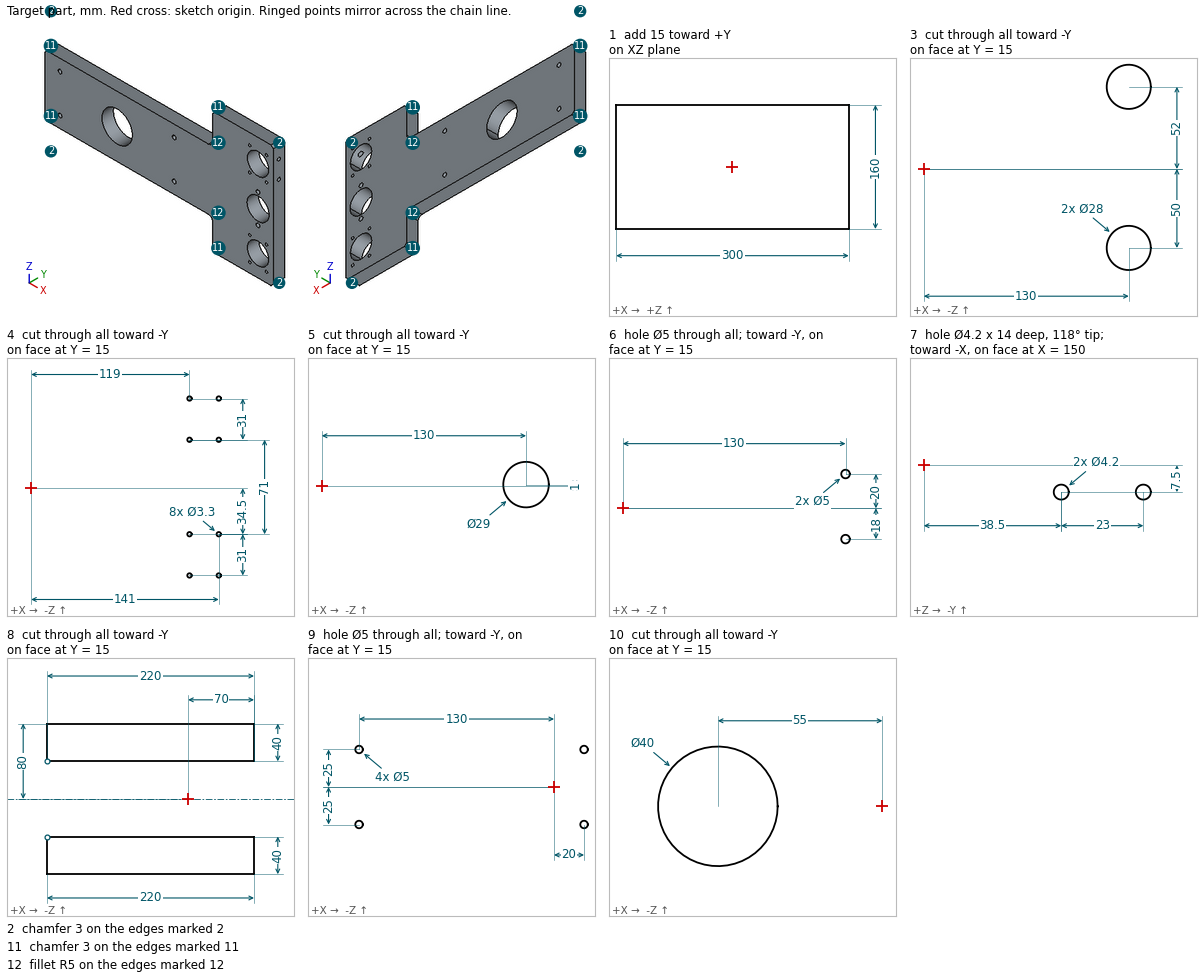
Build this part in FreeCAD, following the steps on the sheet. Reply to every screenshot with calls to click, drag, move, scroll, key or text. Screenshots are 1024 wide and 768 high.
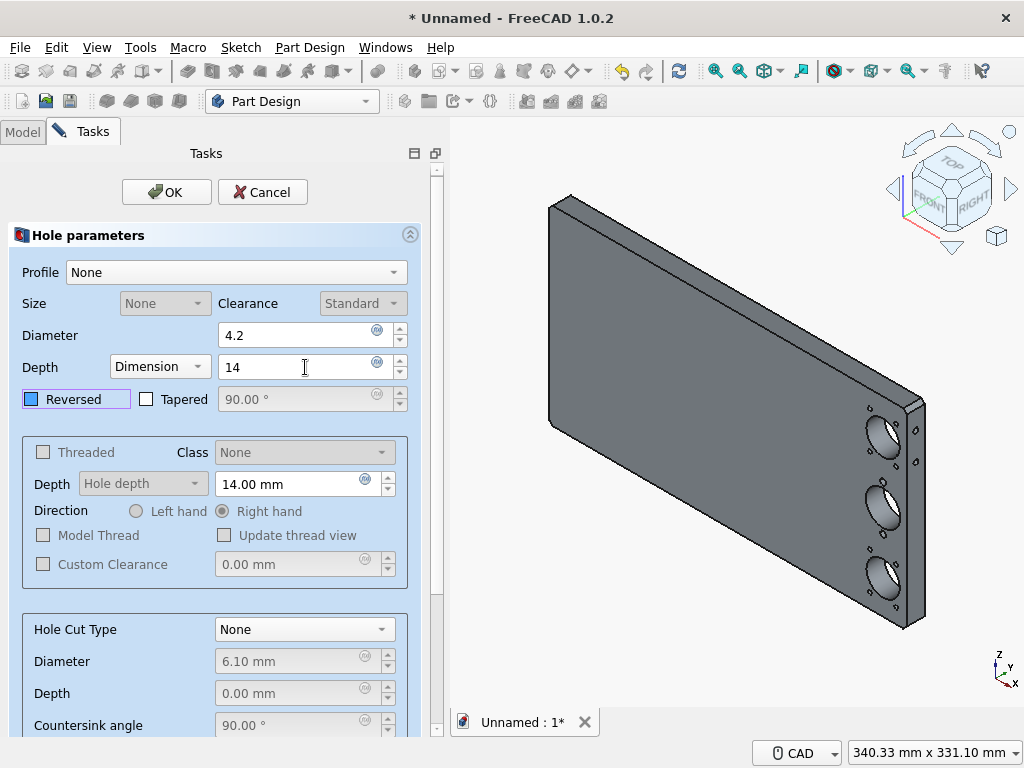
click(167, 192)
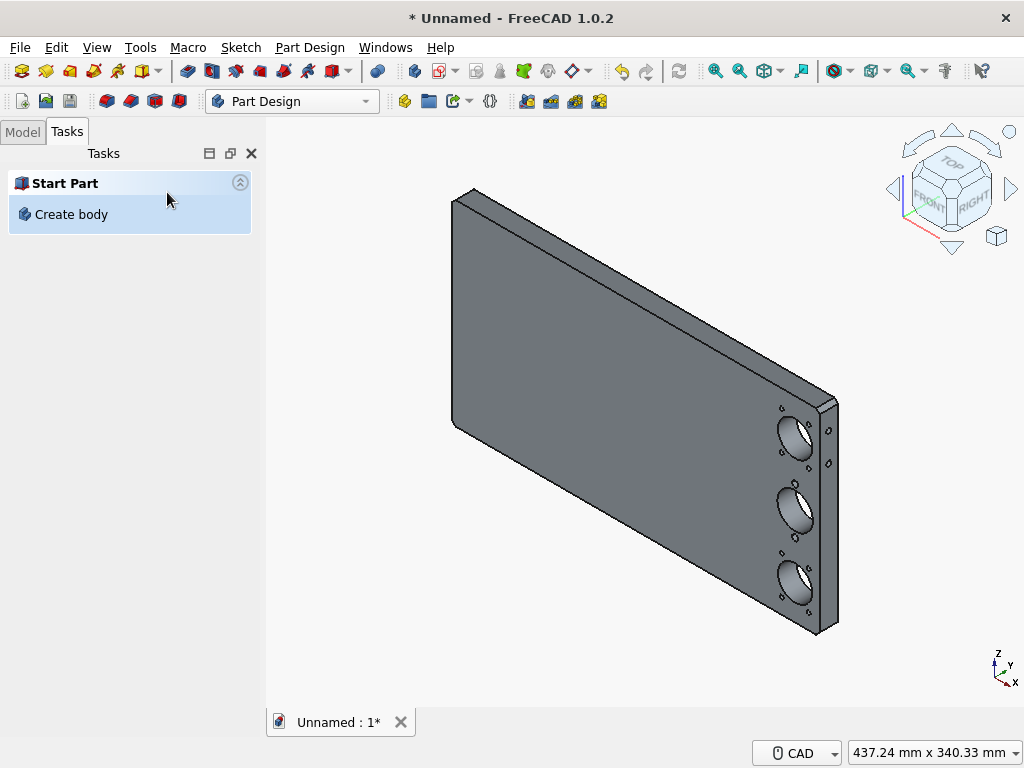
key(4)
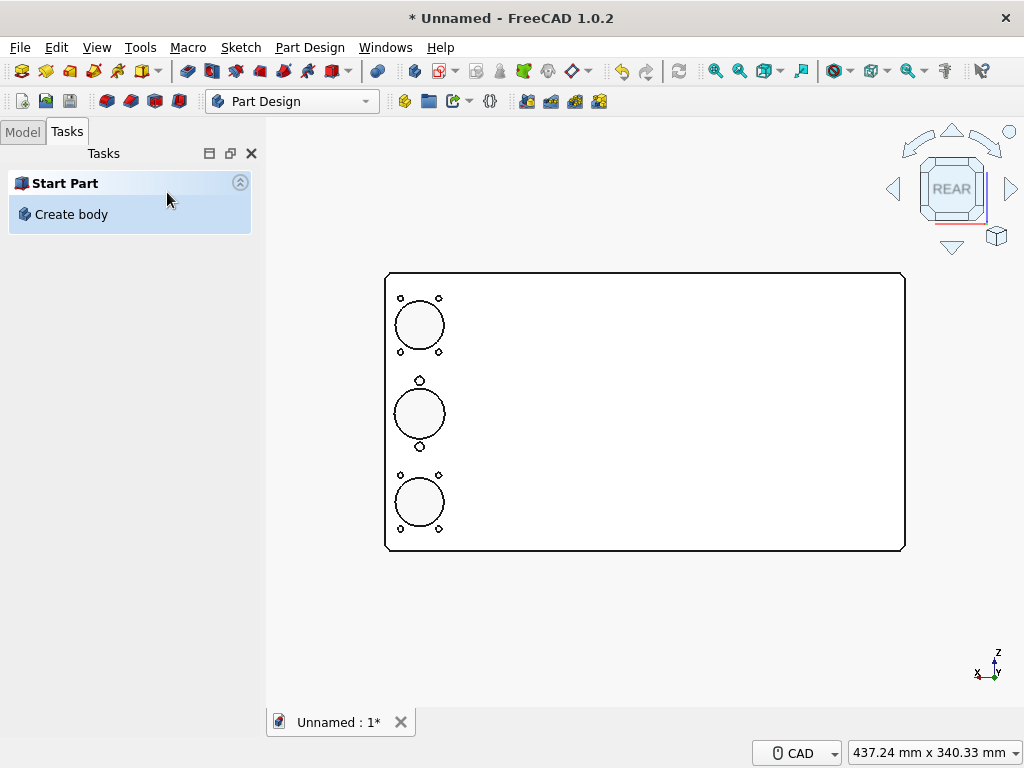
click(645, 411)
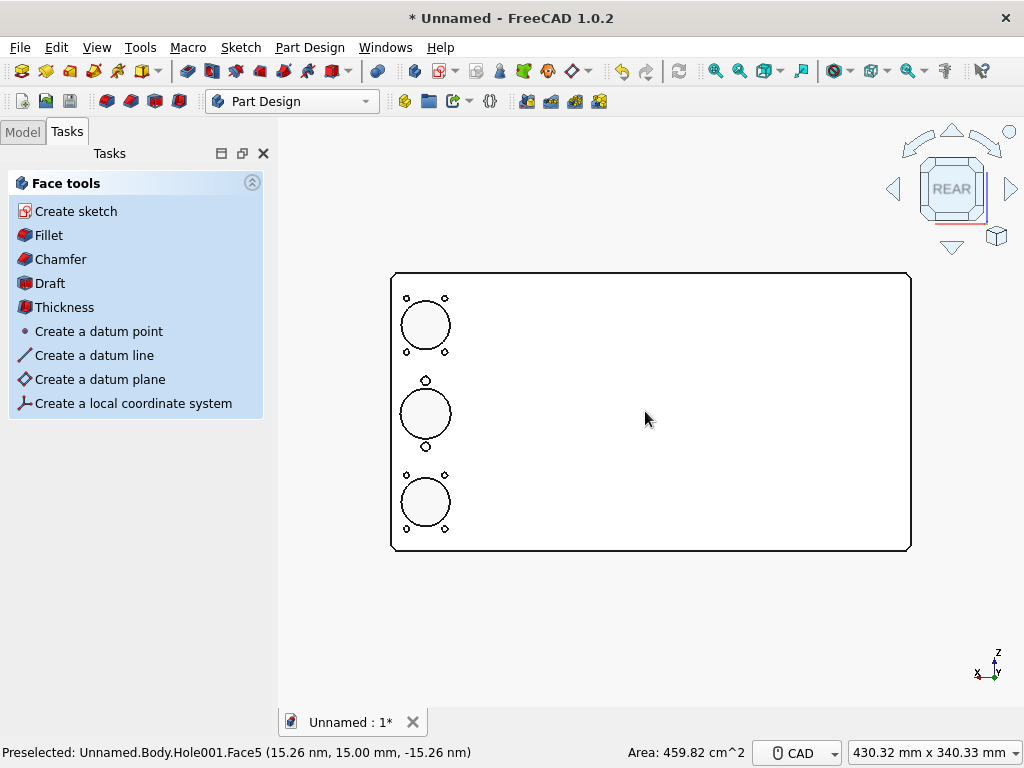
click(440, 72)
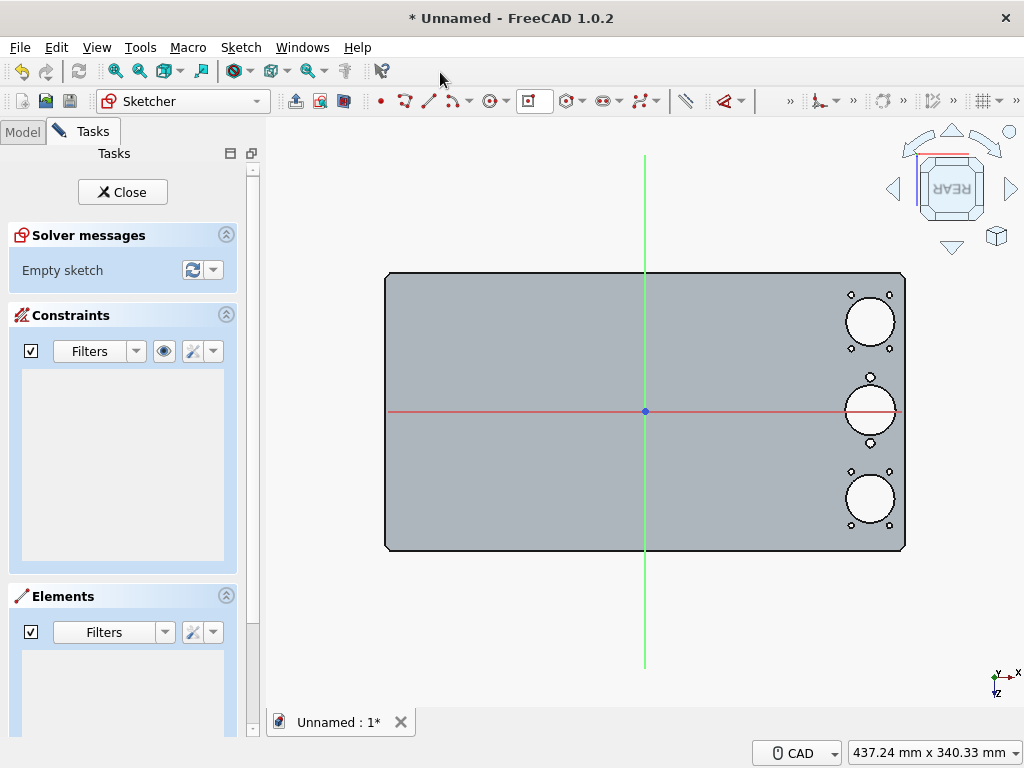
click(548, 102)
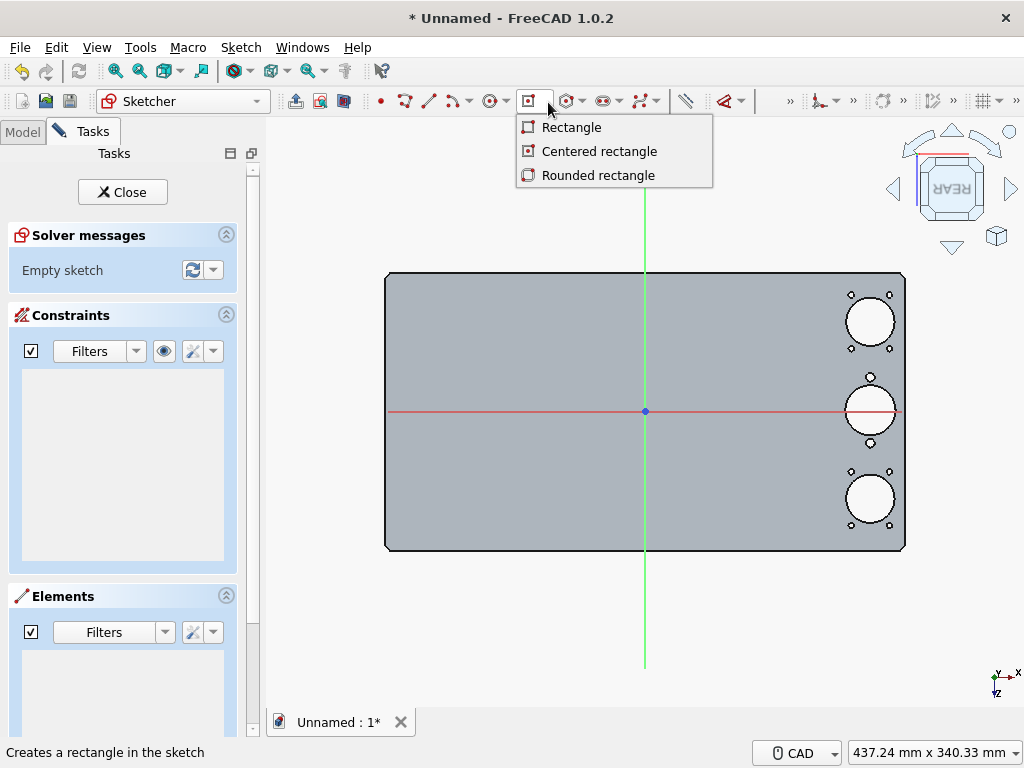
click(614, 127)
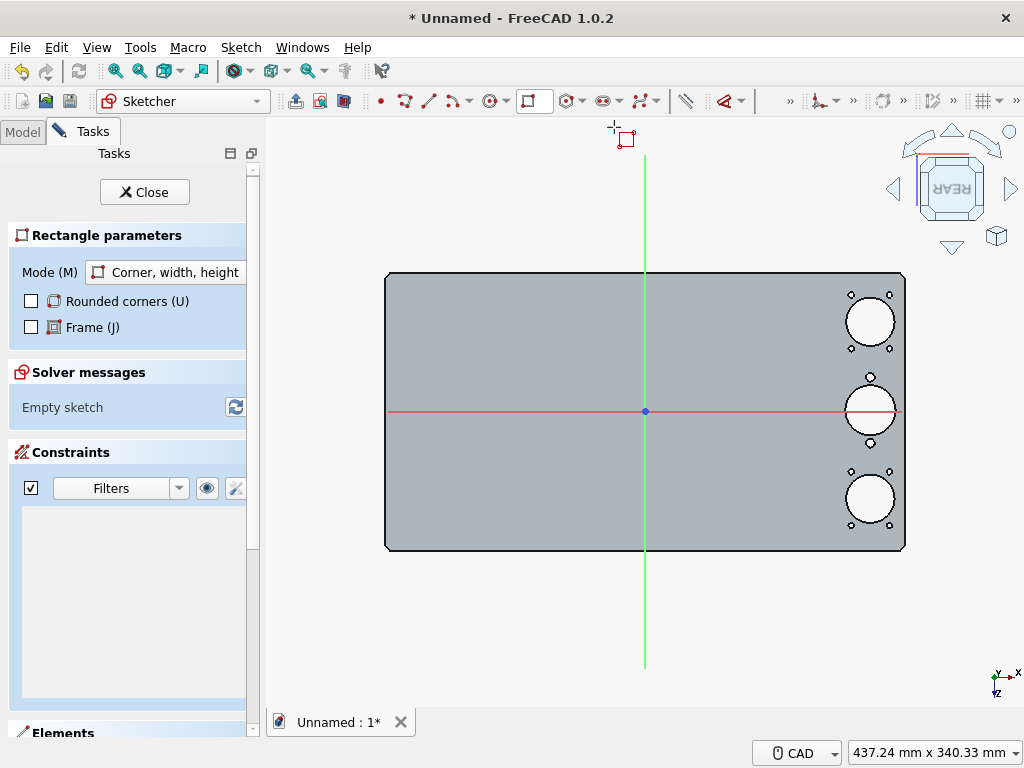
click(385, 273)
move(766, 343)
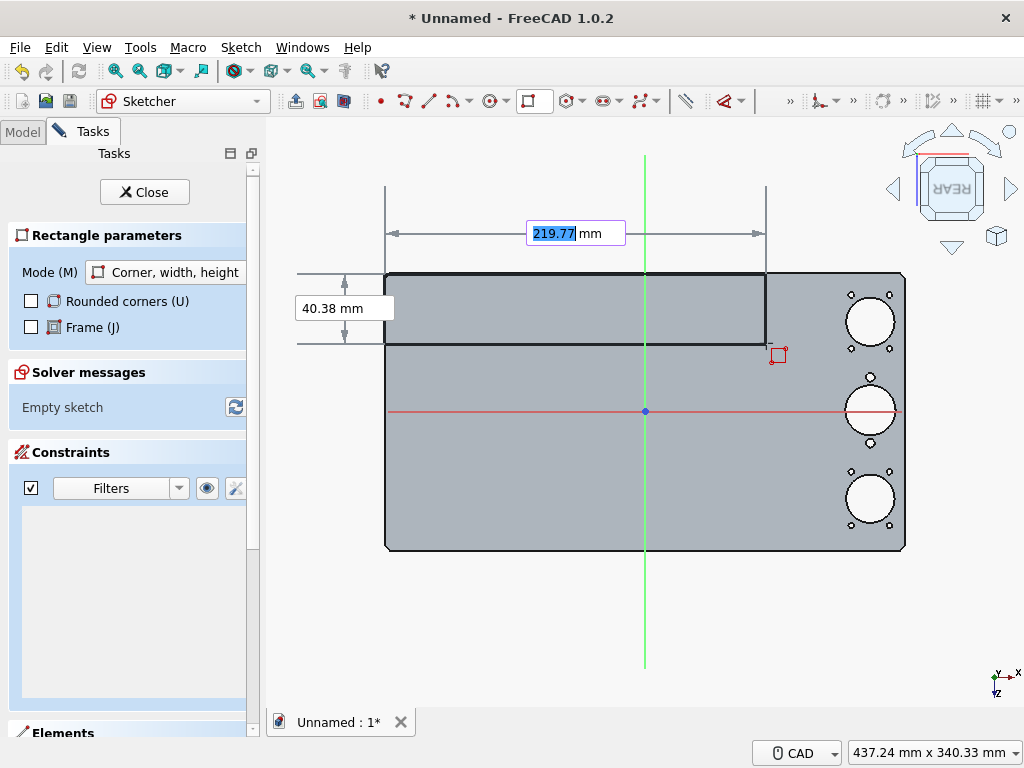
text(220)
key(Tab)
text(40)
key(Return)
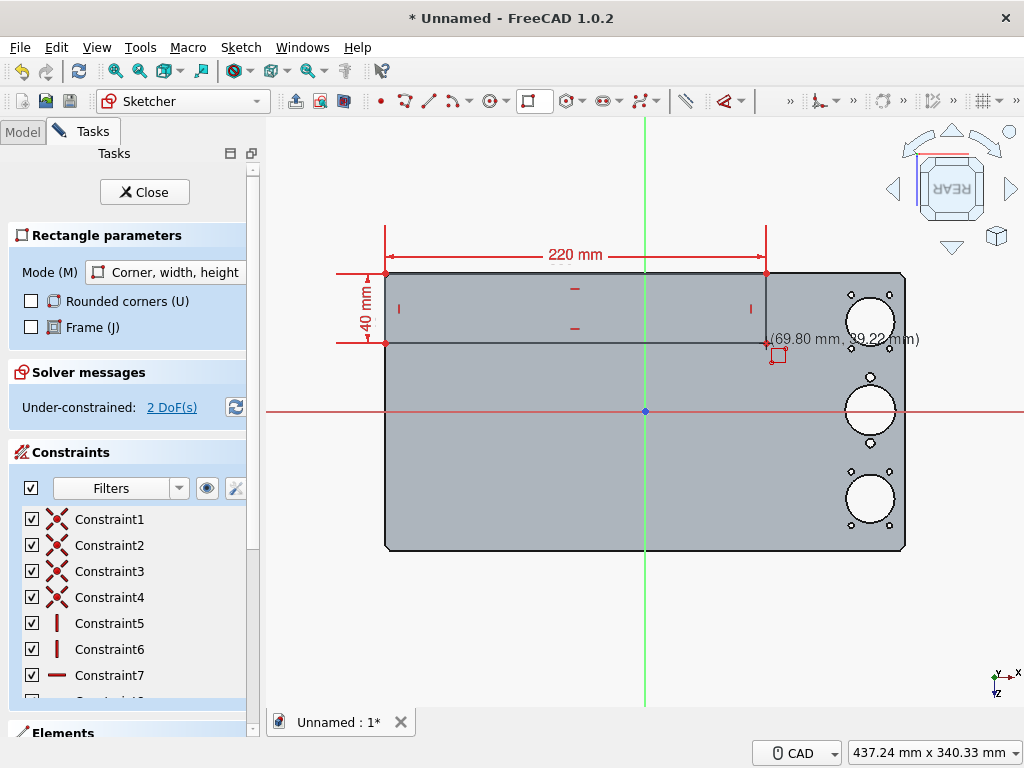
click(385, 481)
move(766, 551)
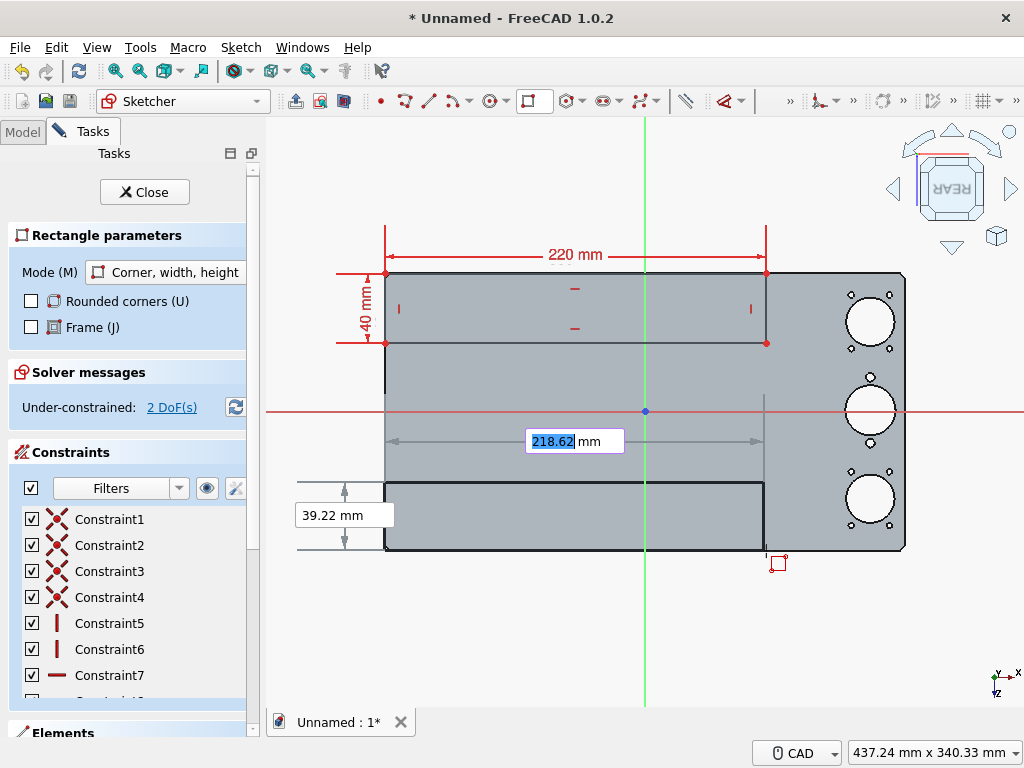
text(220)
key(Tab)
text(40)
key(Return)
key(Escape)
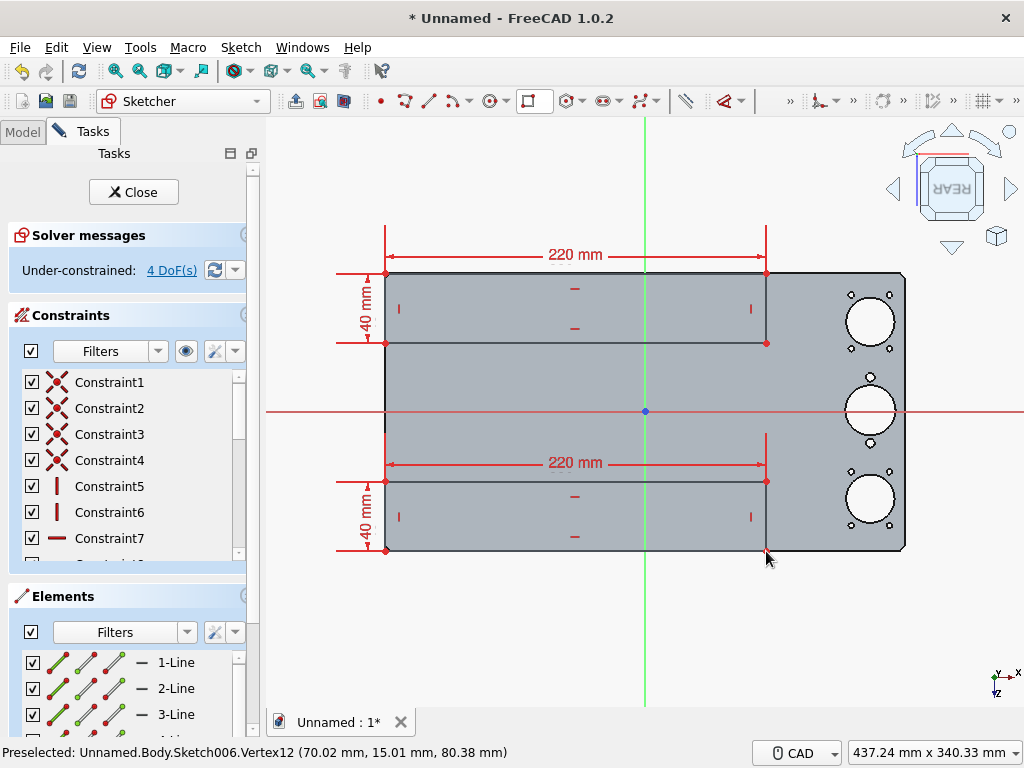
click(385, 343)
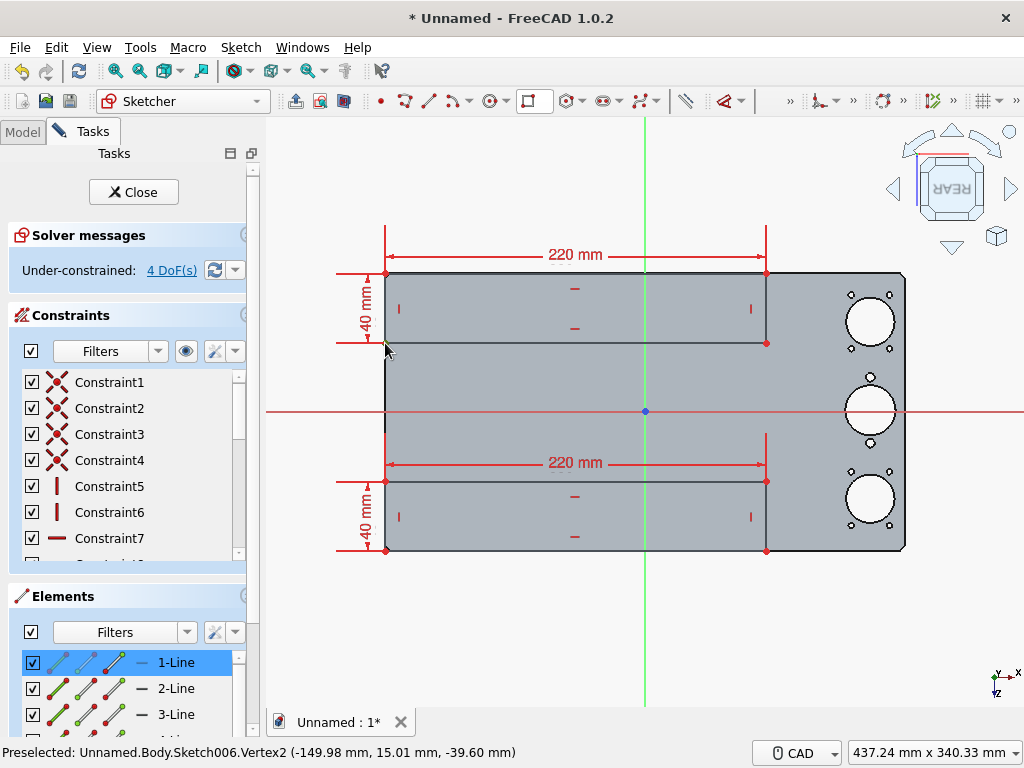
click(385, 482)